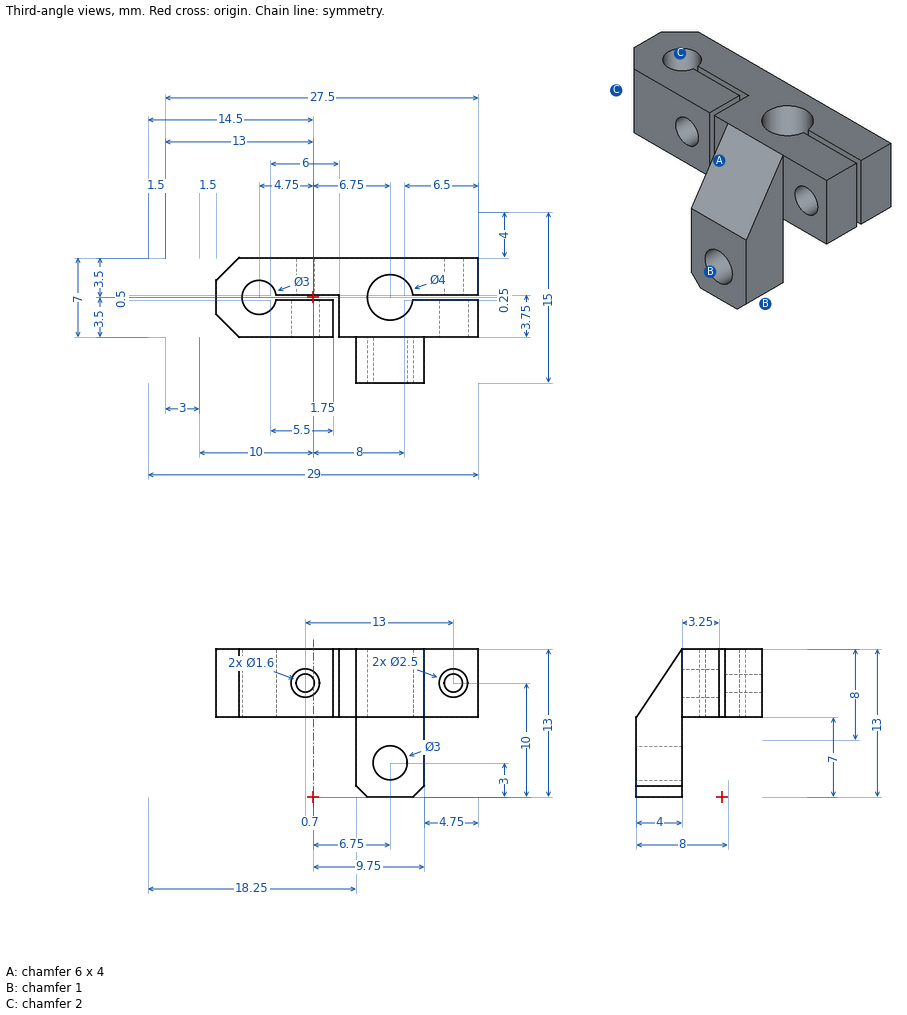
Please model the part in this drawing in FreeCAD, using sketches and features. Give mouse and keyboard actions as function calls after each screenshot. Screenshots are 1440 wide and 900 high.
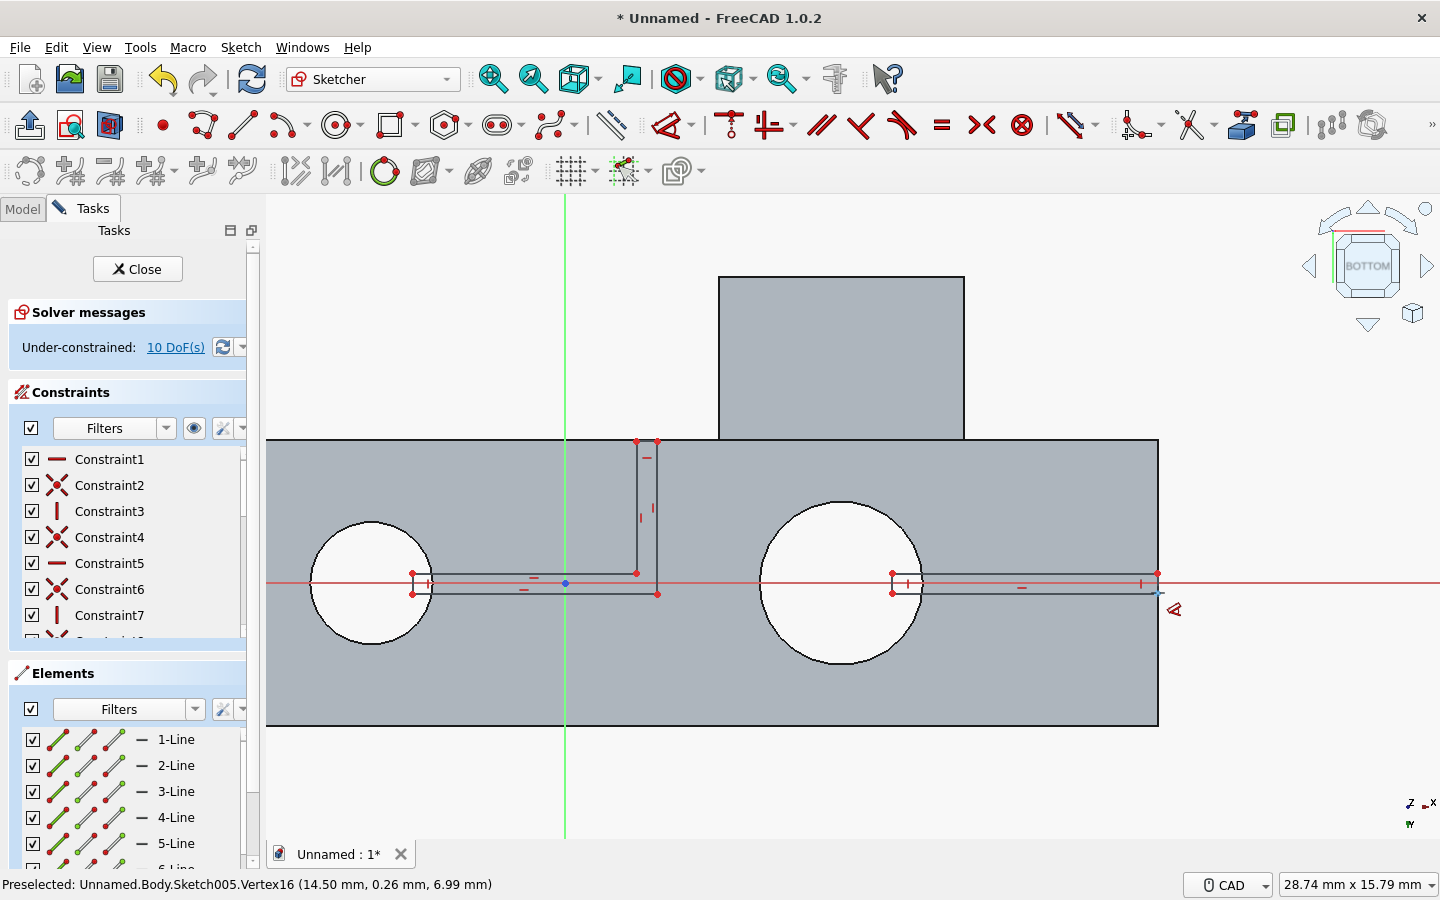
scroll(486, 594, up, 2)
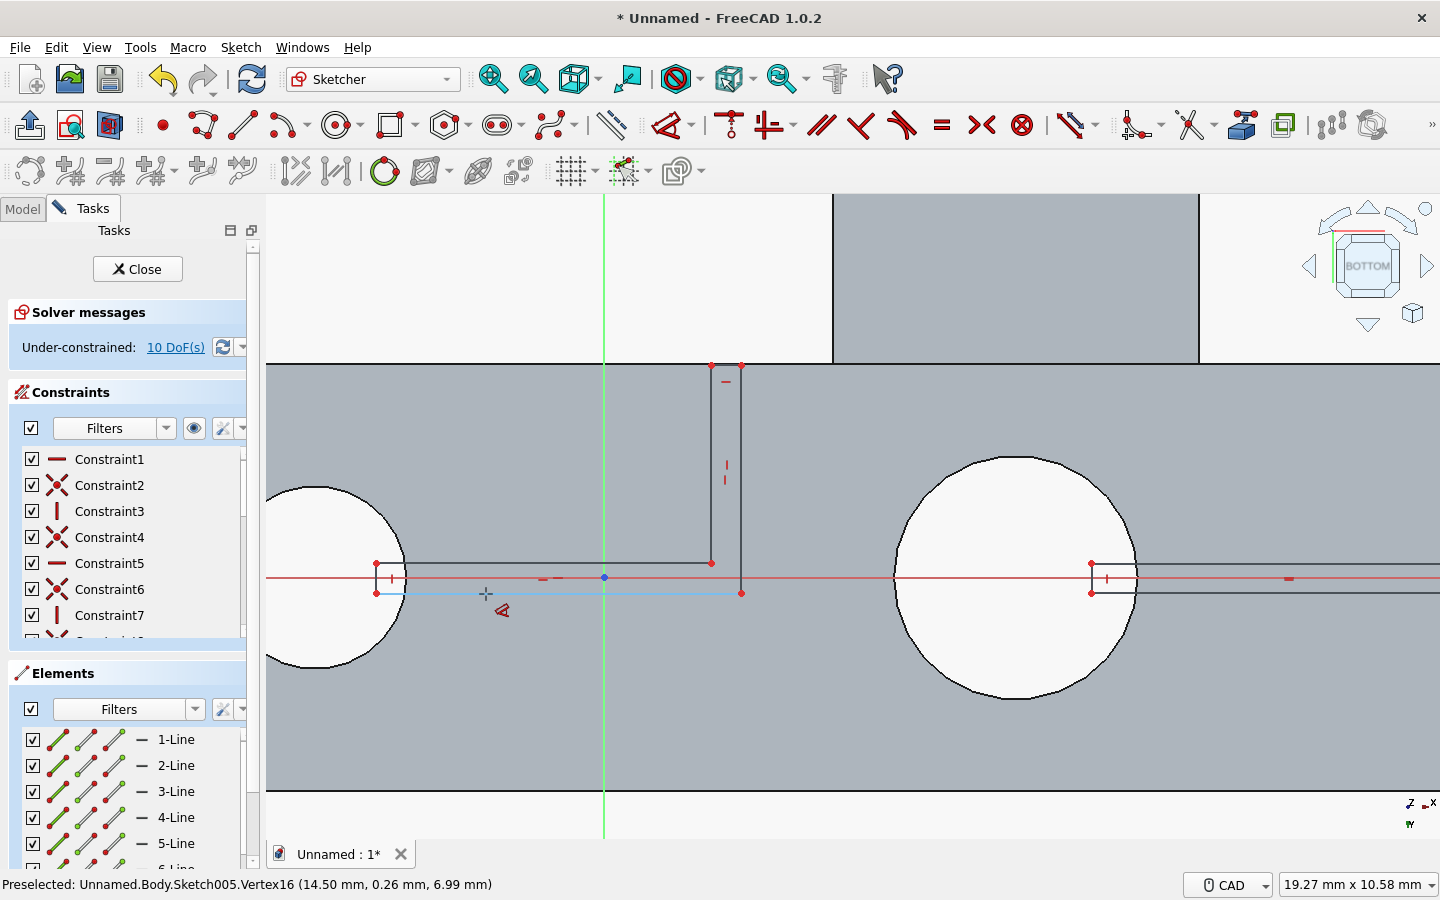
click(486, 594)
click(559, 628)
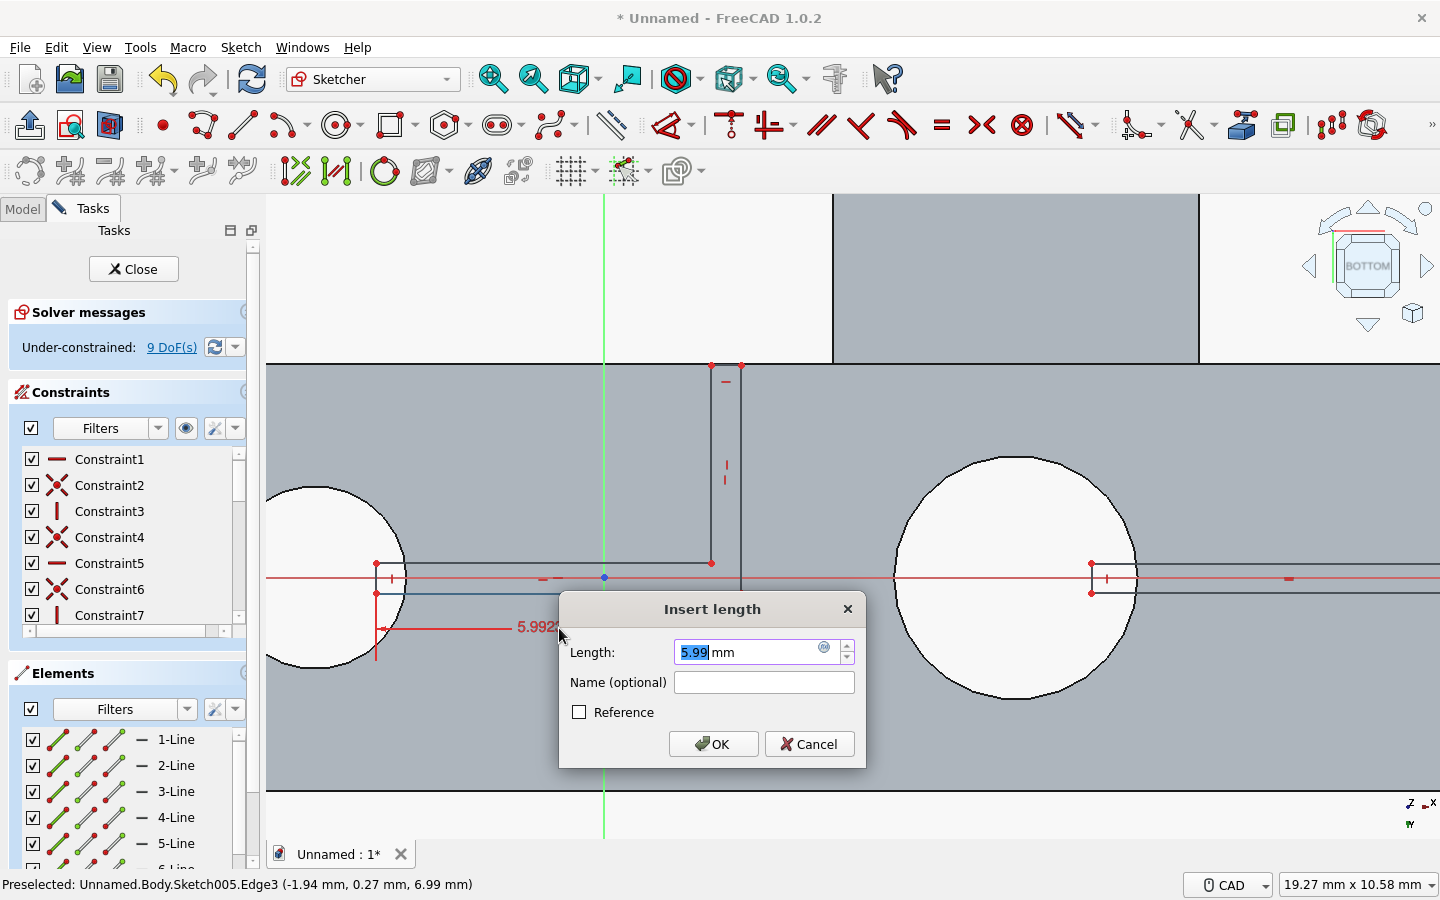
text(6)
key(Return)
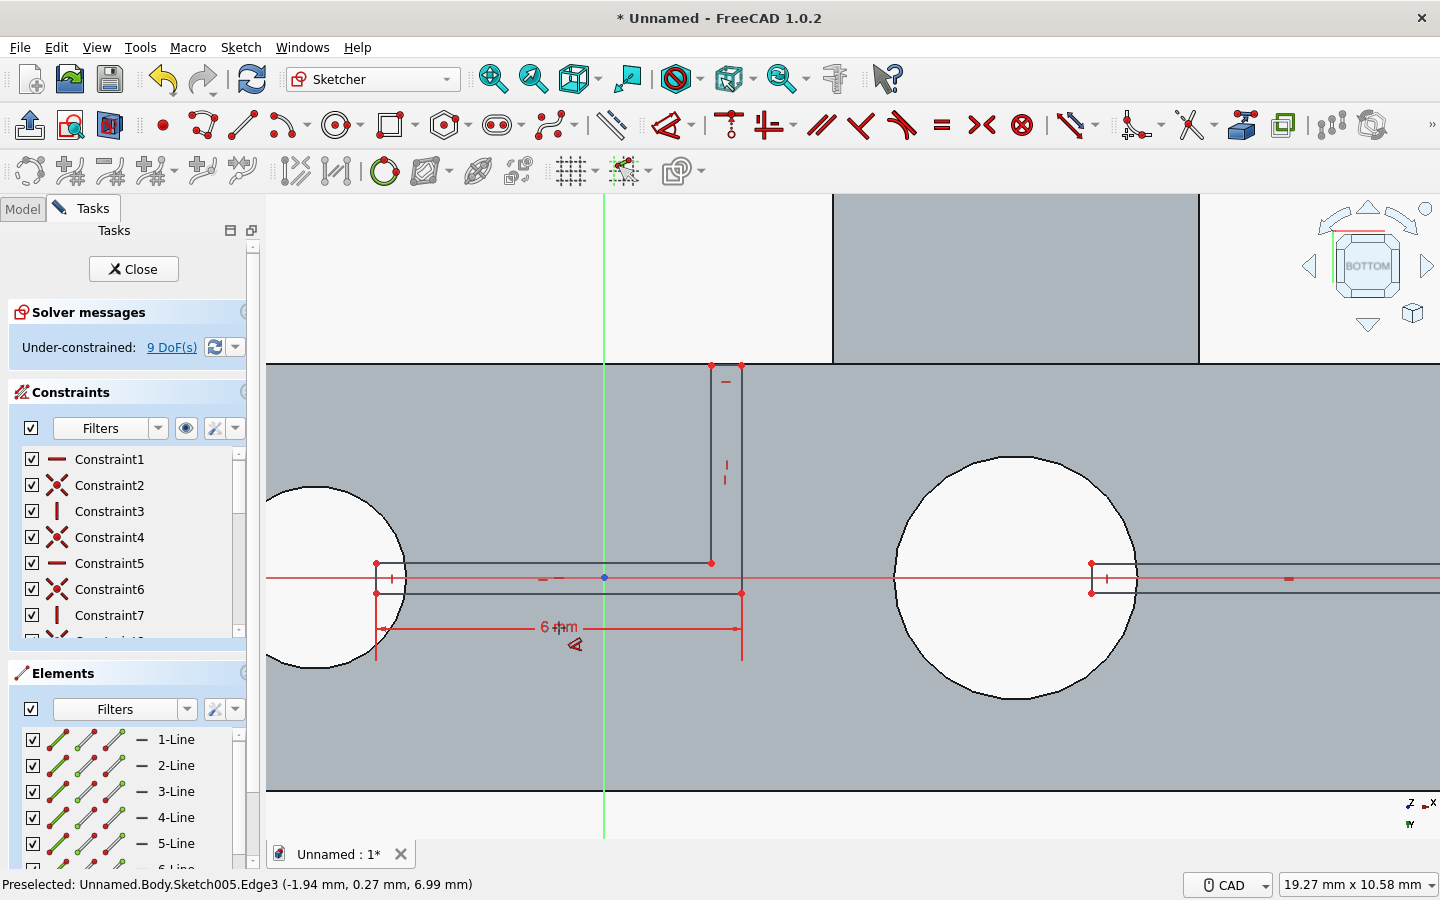
click(1092, 564)
click(848, 612)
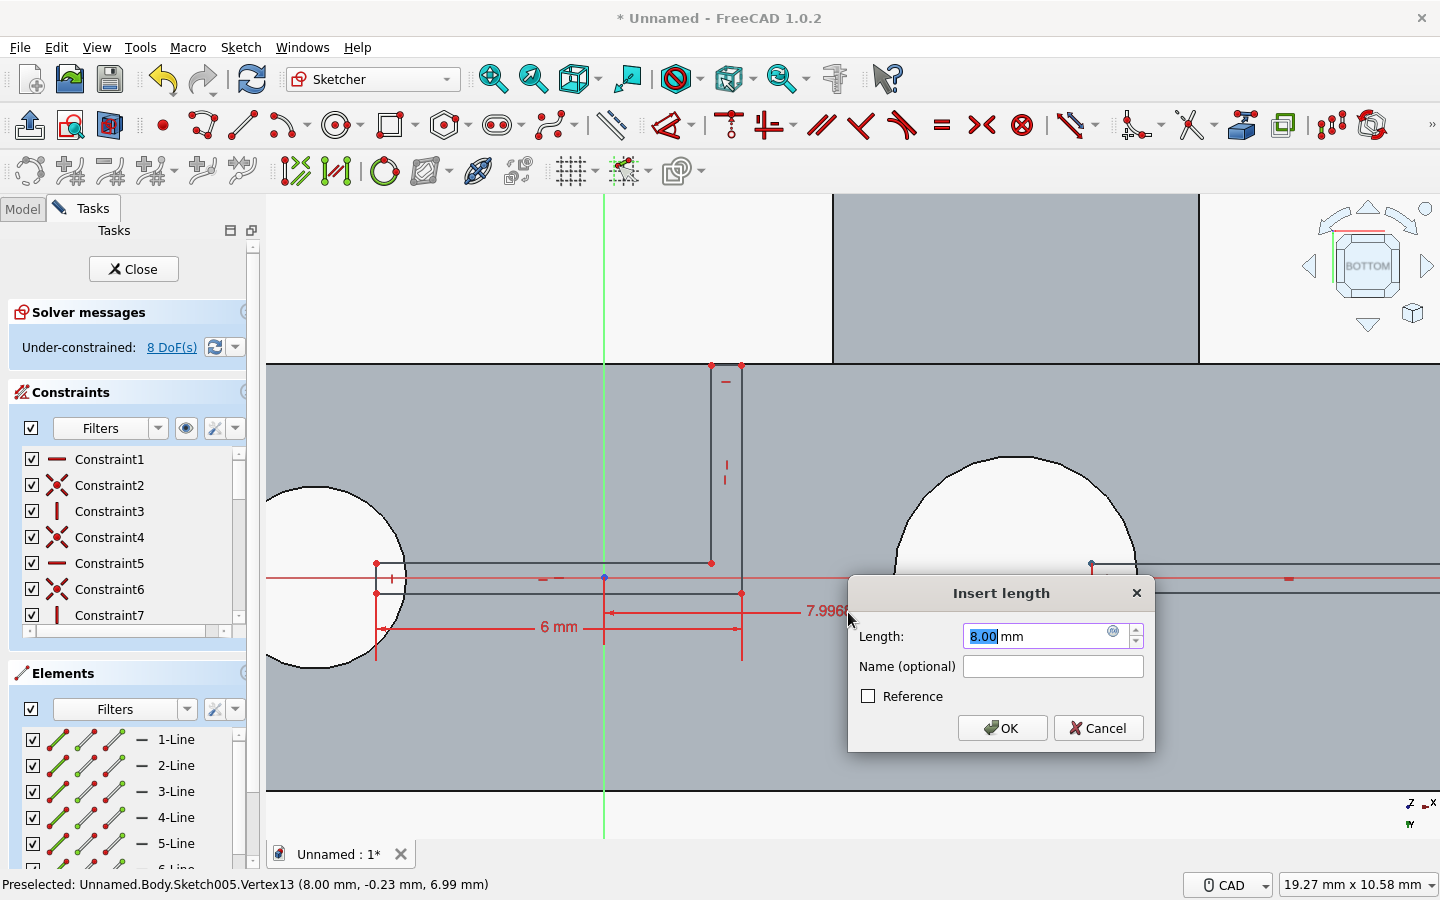
text(8)
key(Return)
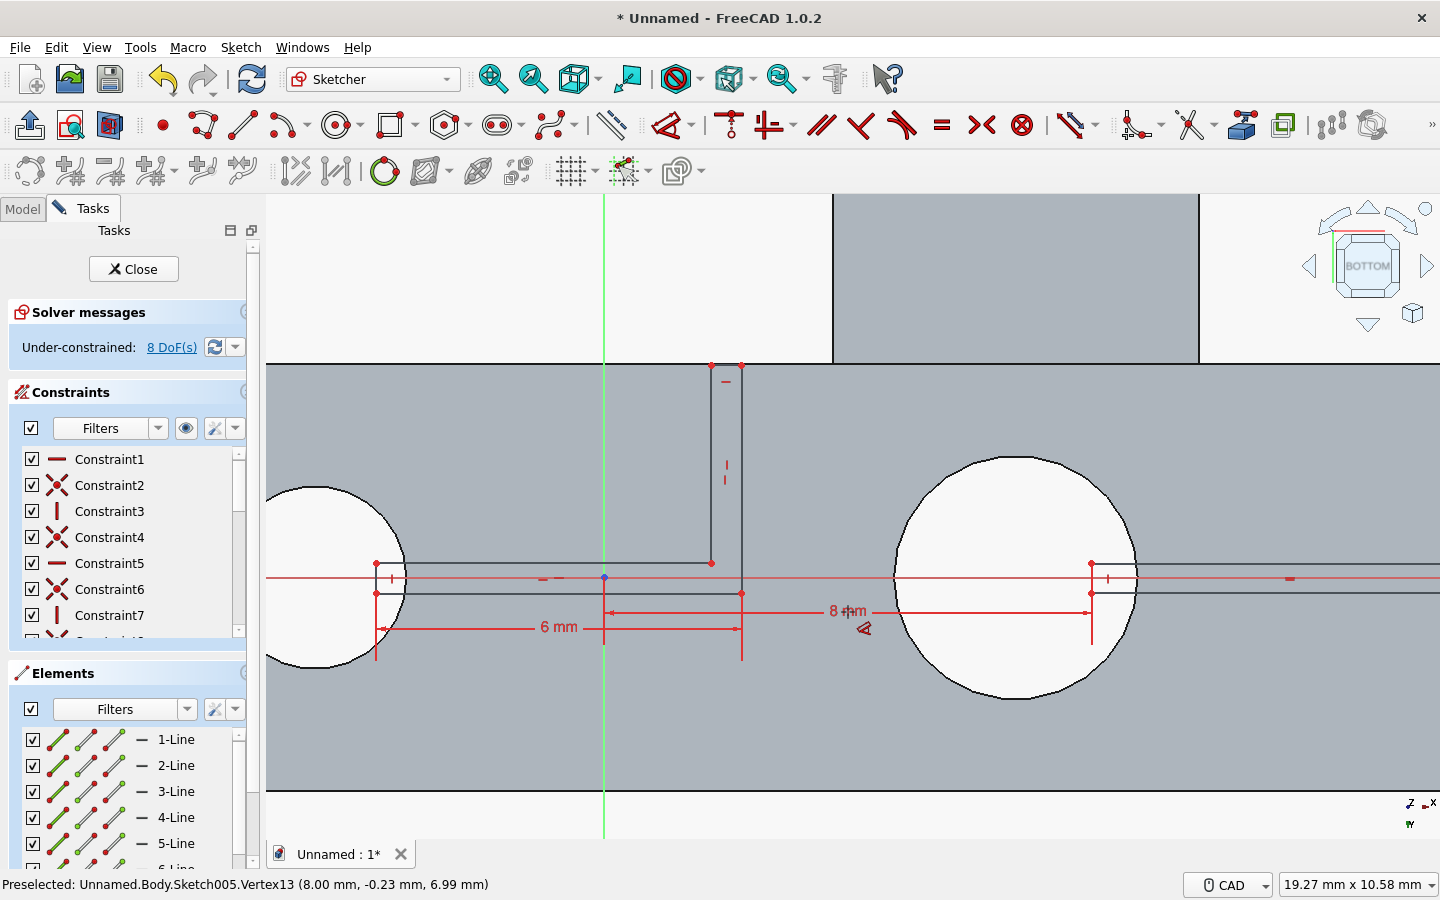
click(477, 563)
click(544, 529)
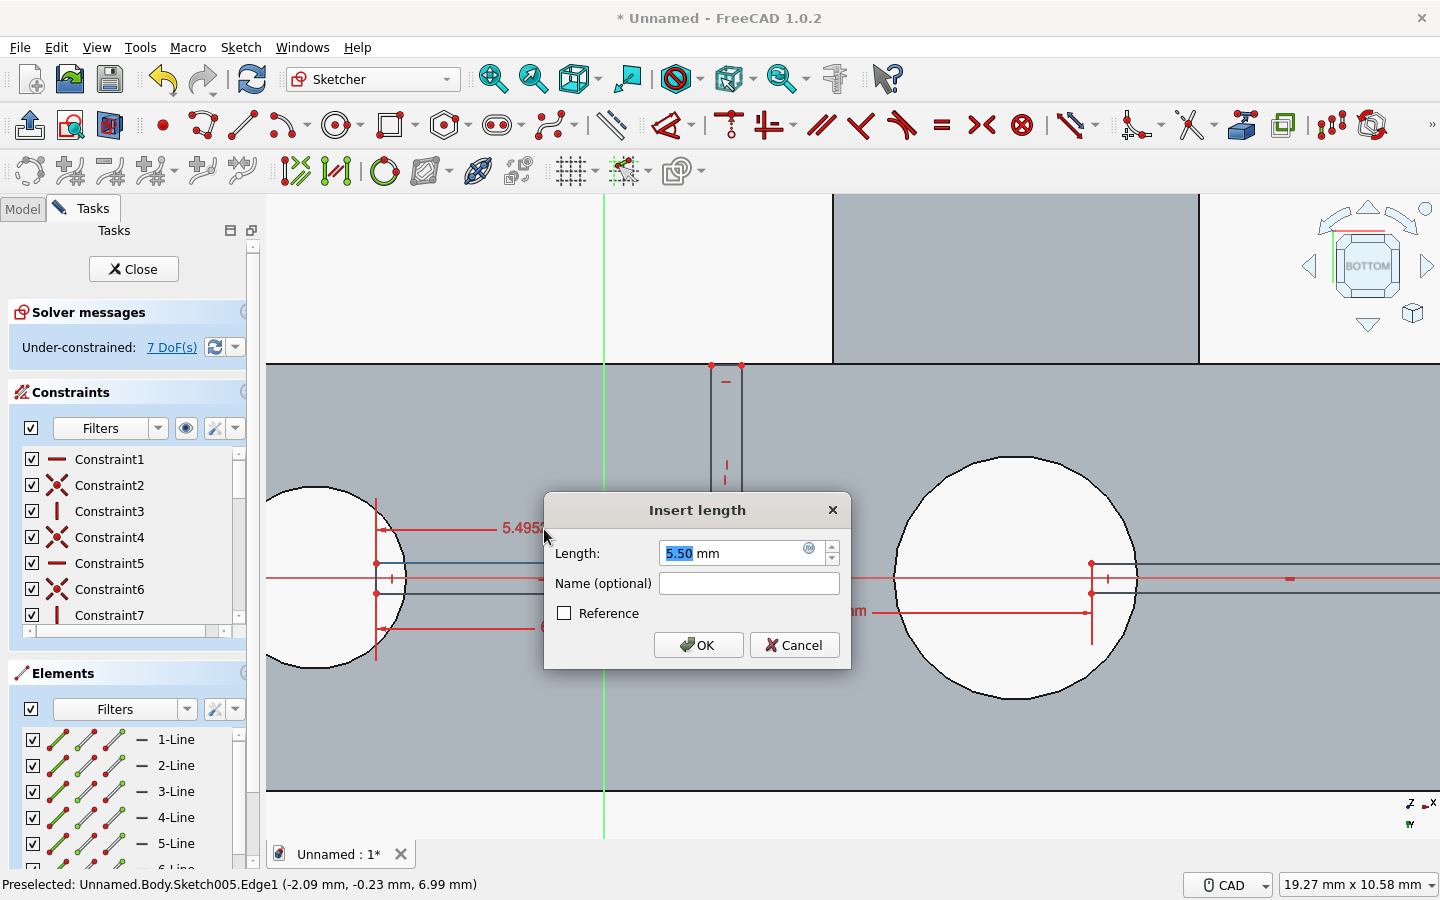
text(5.5)
key(Return)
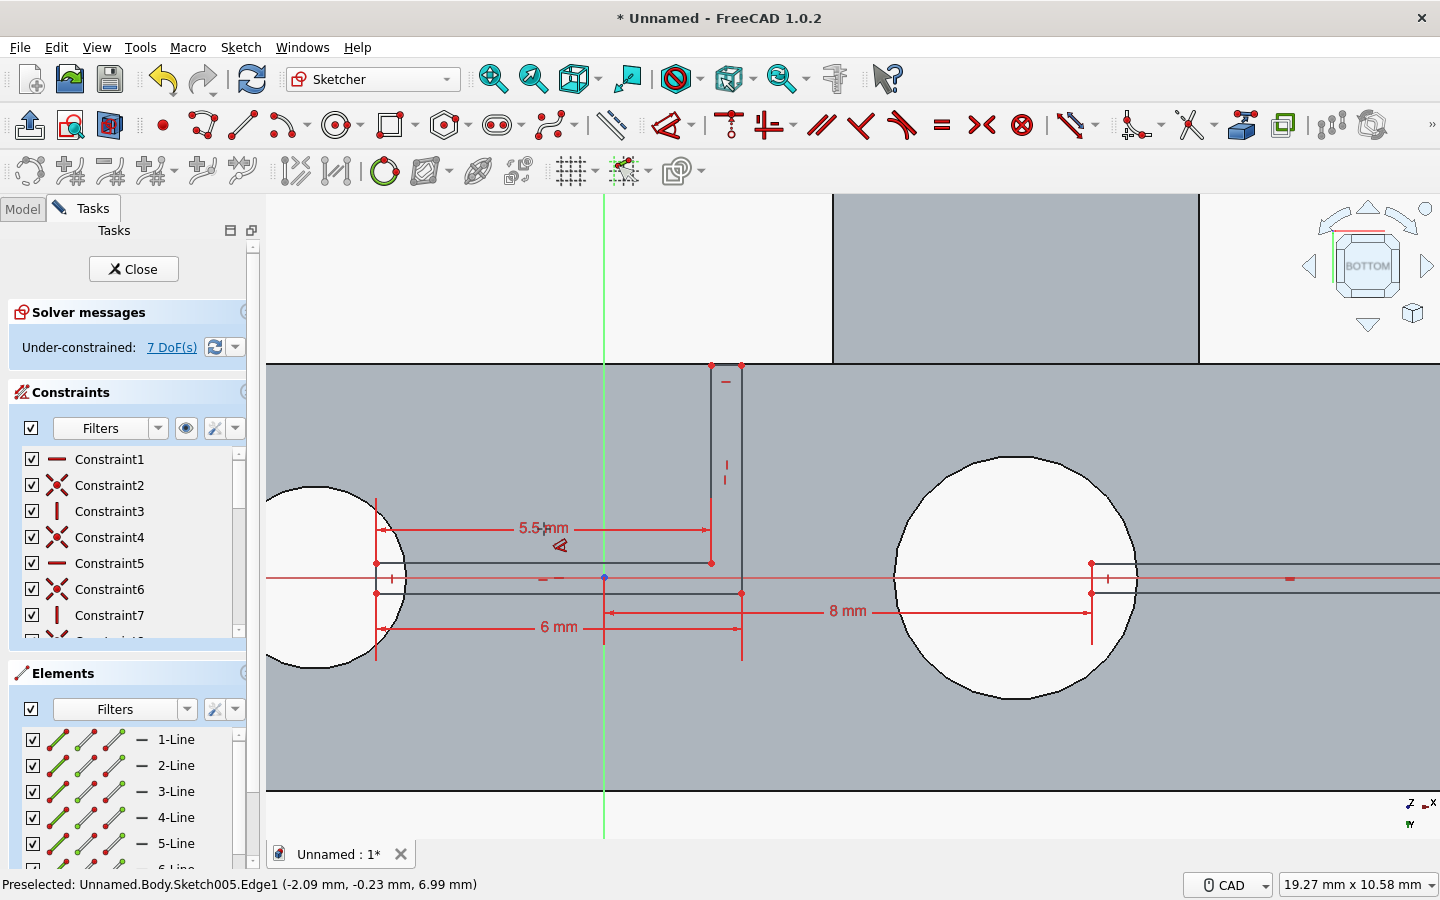
scroll(376, 576, up, 2)